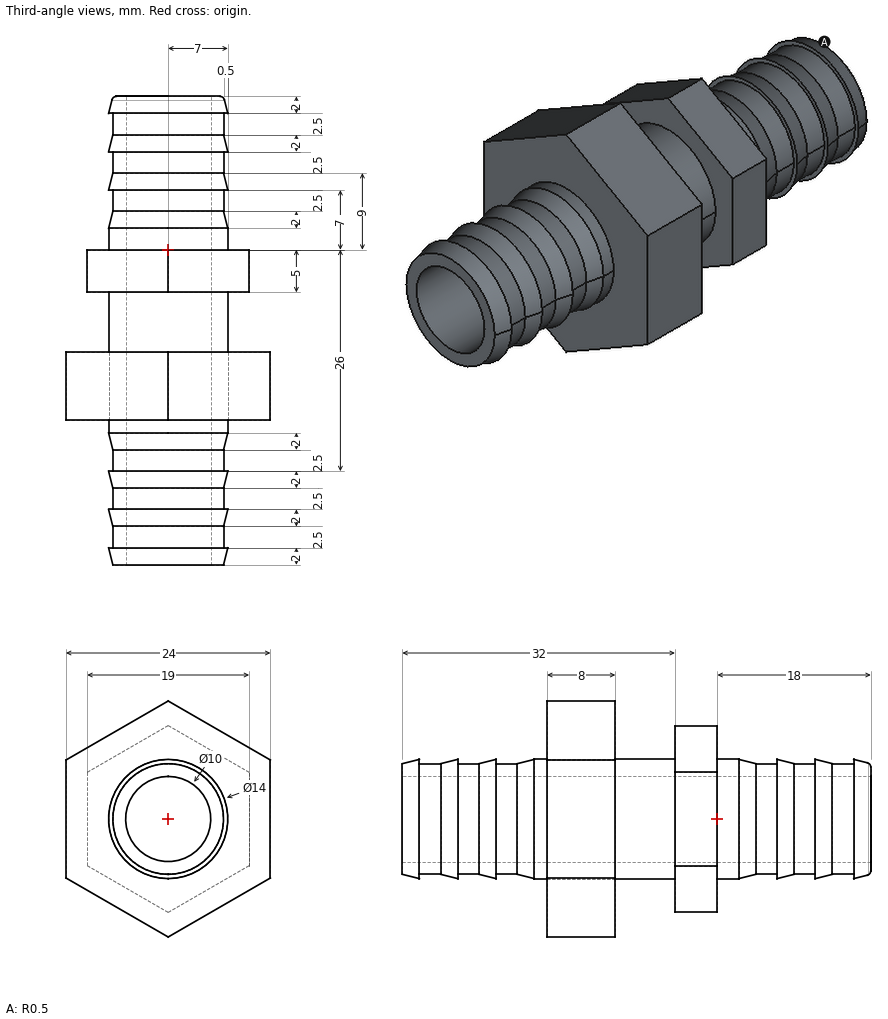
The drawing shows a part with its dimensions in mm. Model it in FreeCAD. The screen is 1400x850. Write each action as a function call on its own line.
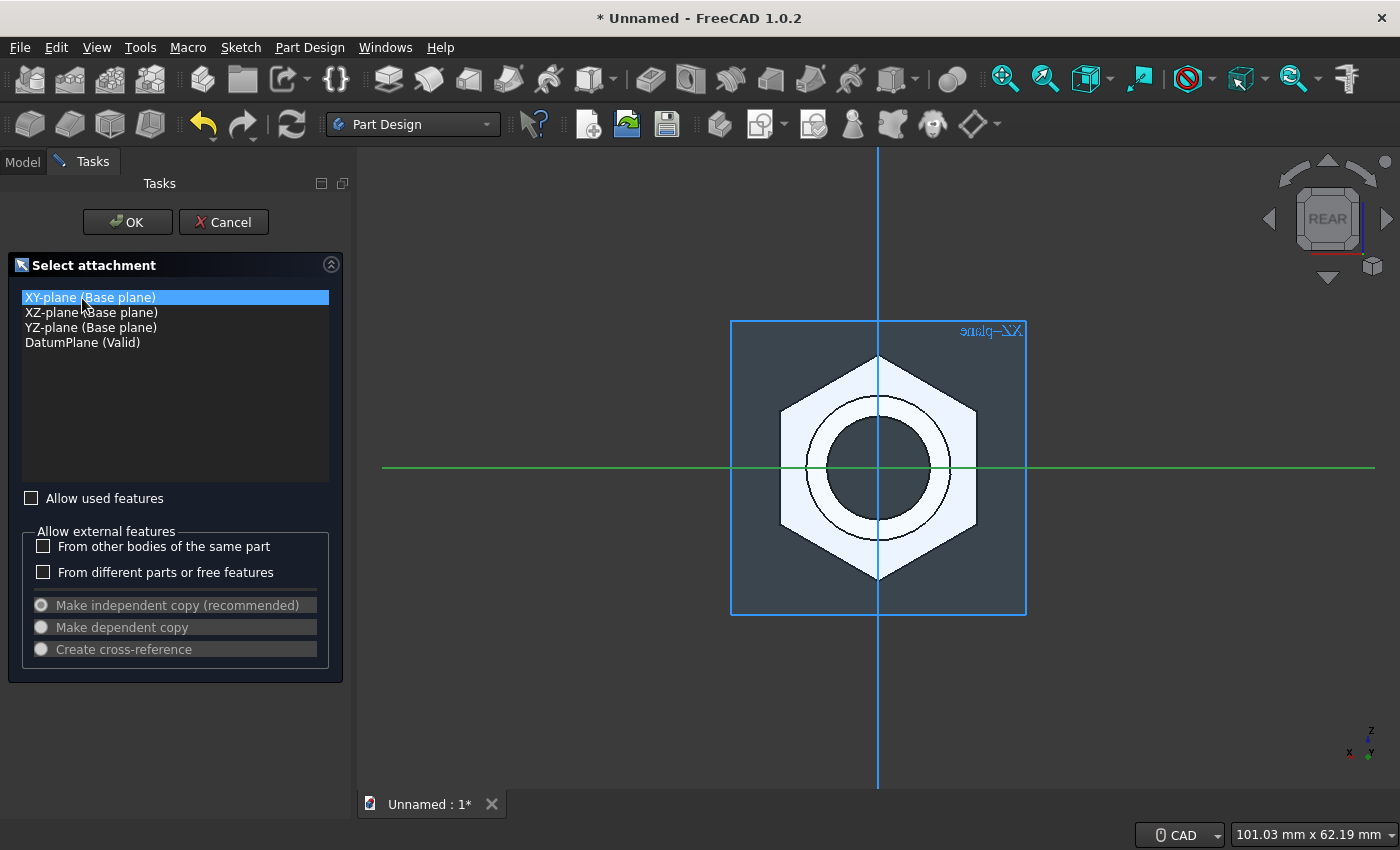
click(128, 222)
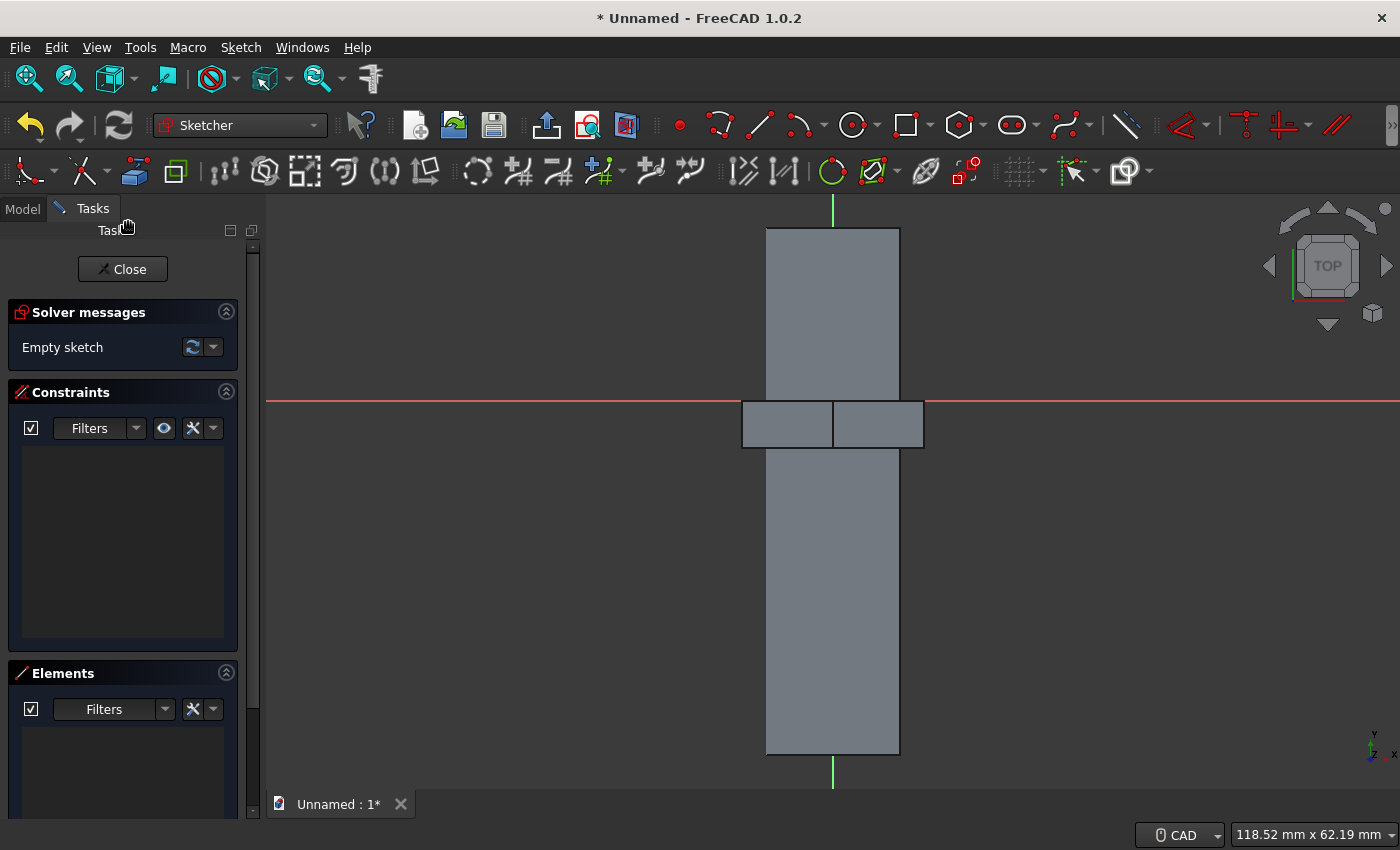
click(628, 126)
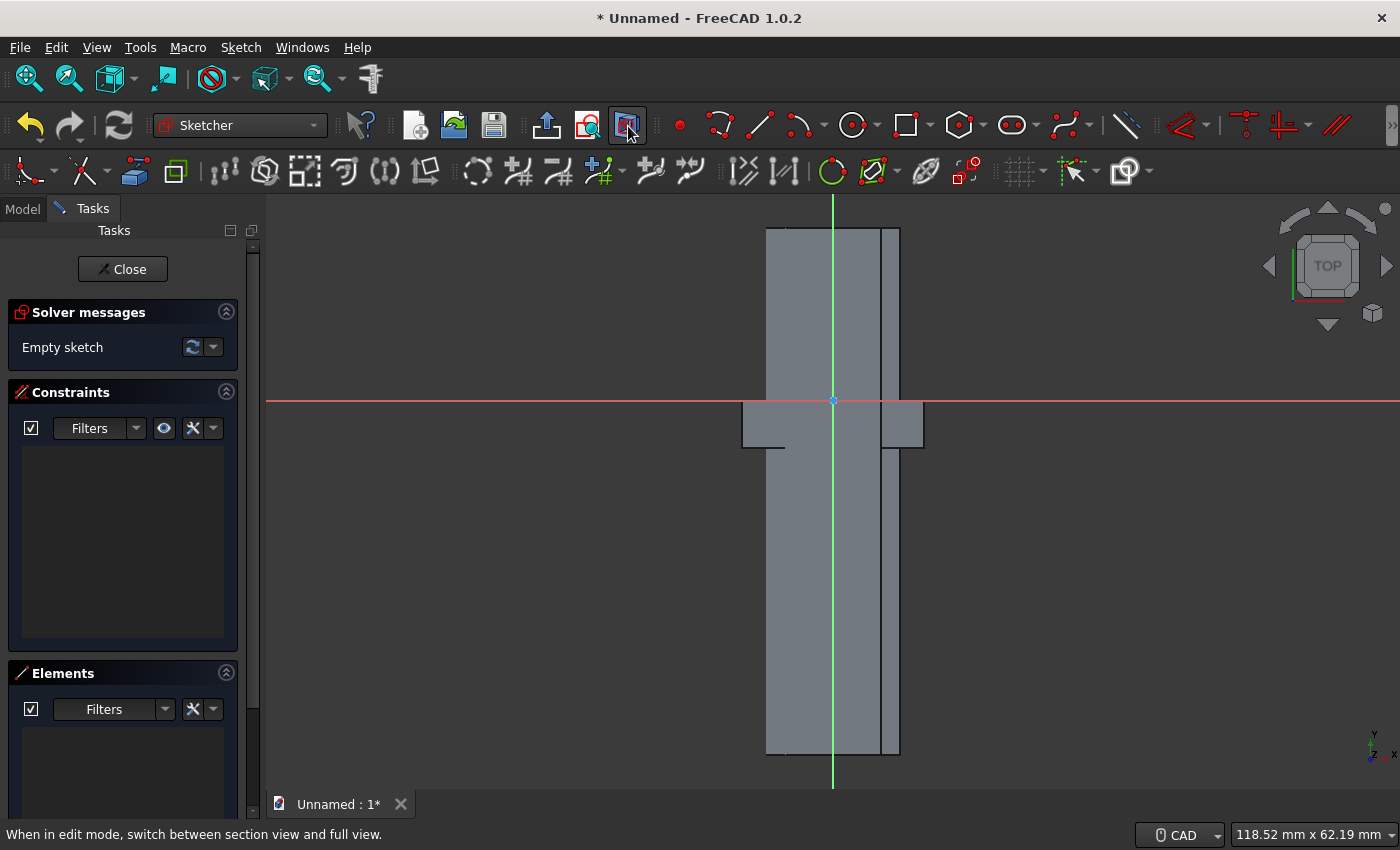
scroll(557, 492, down, 2)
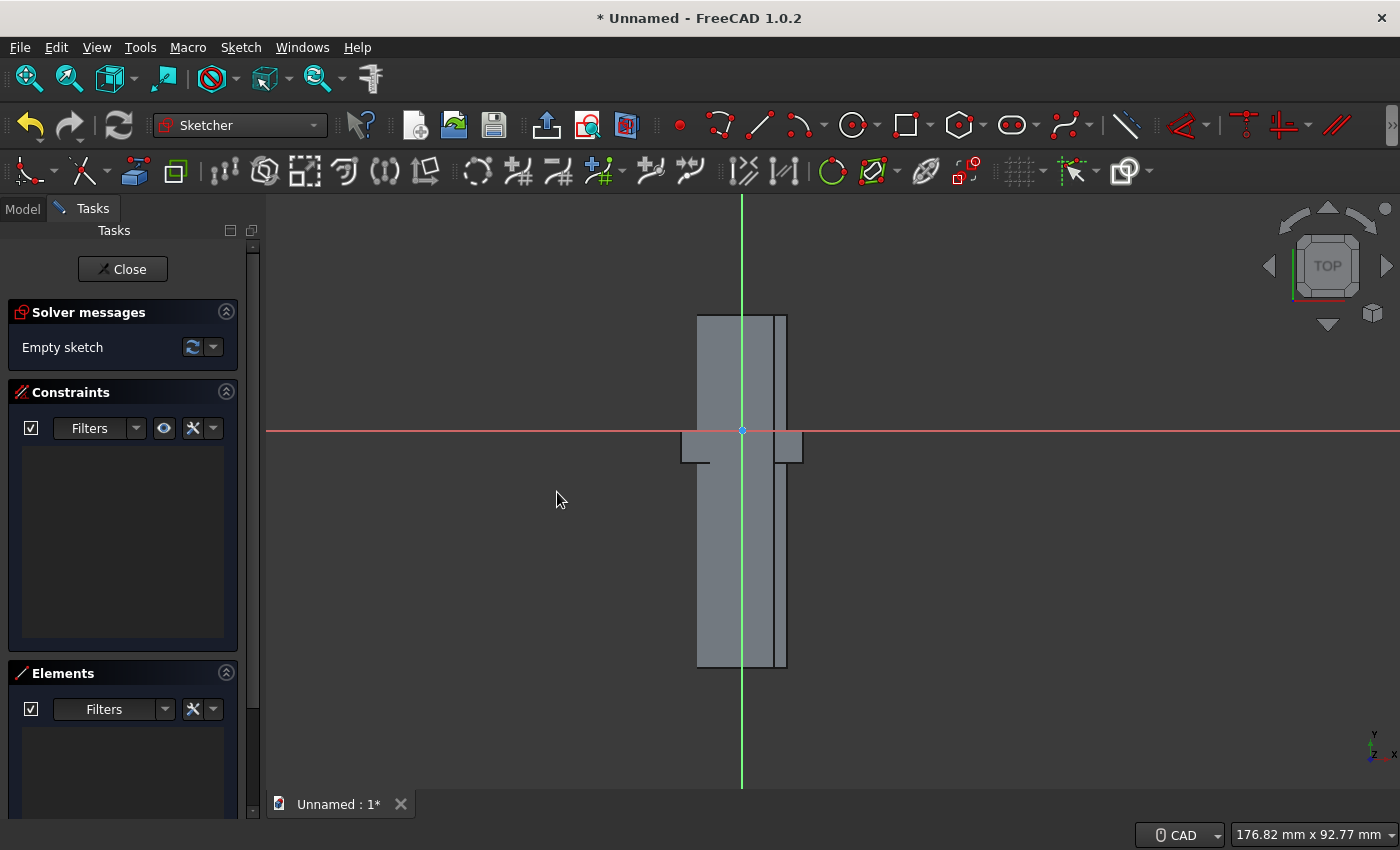
click(720, 126)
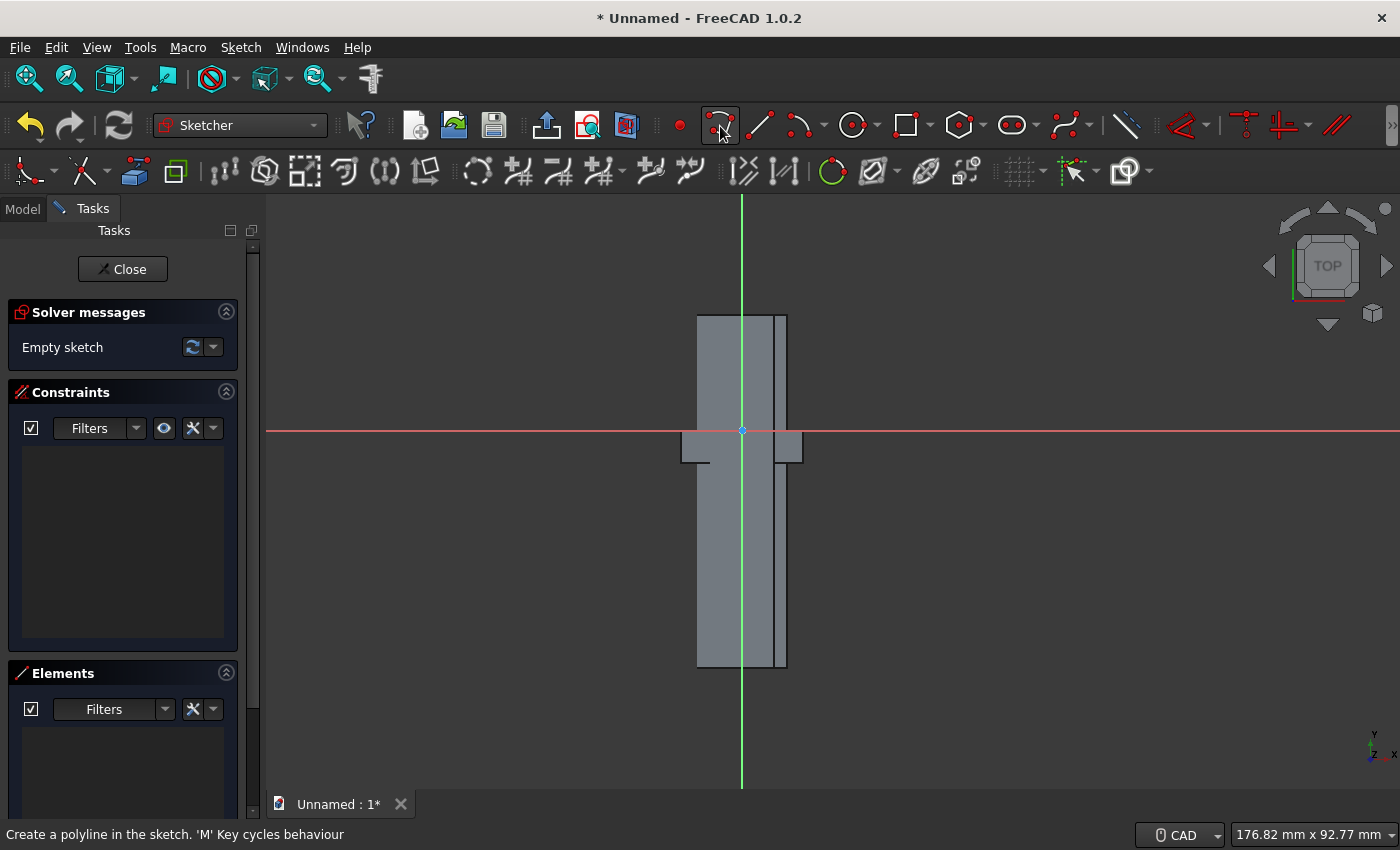
click(787, 415)
click(787, 315)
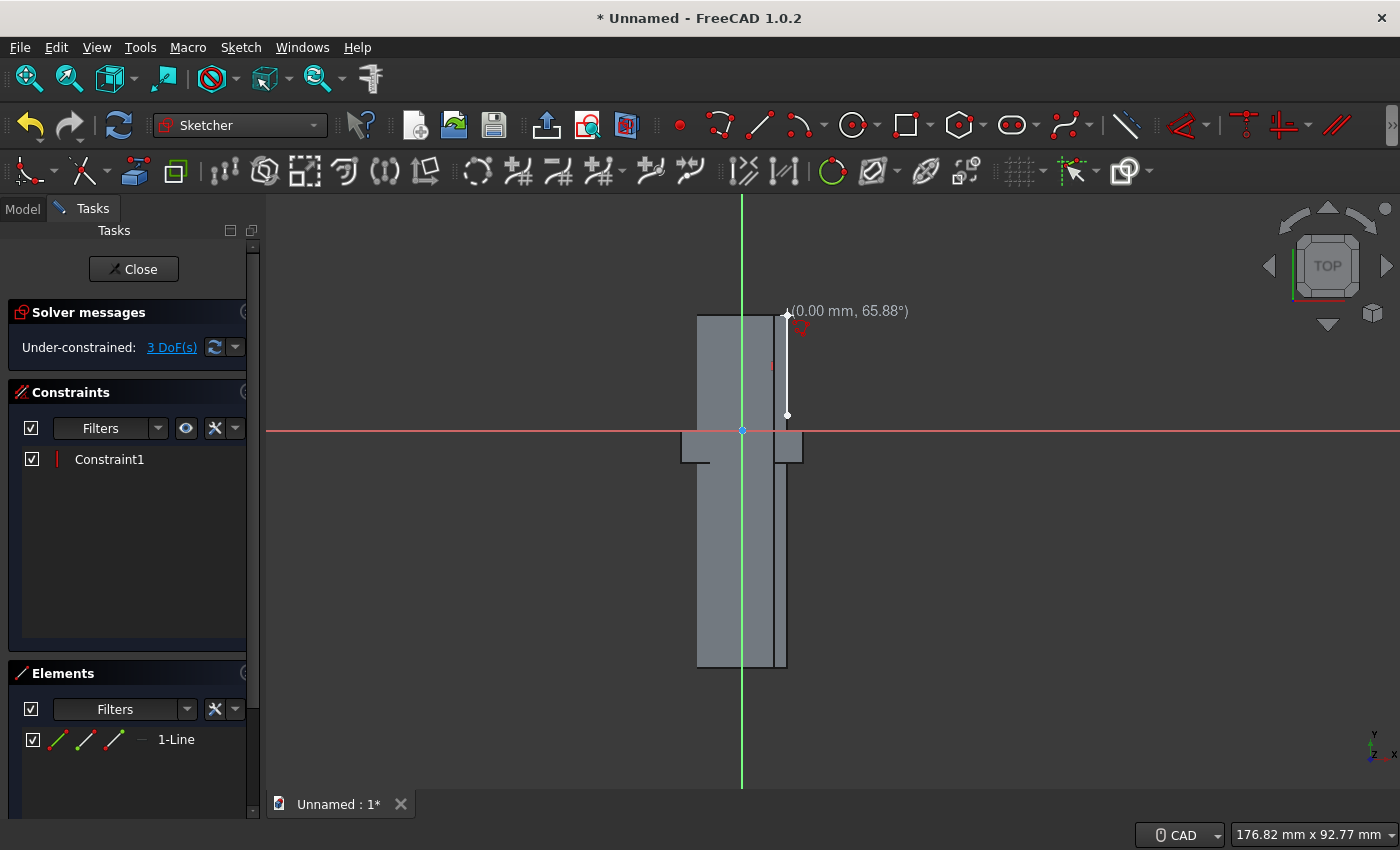
scroll(784, 315, up, 8)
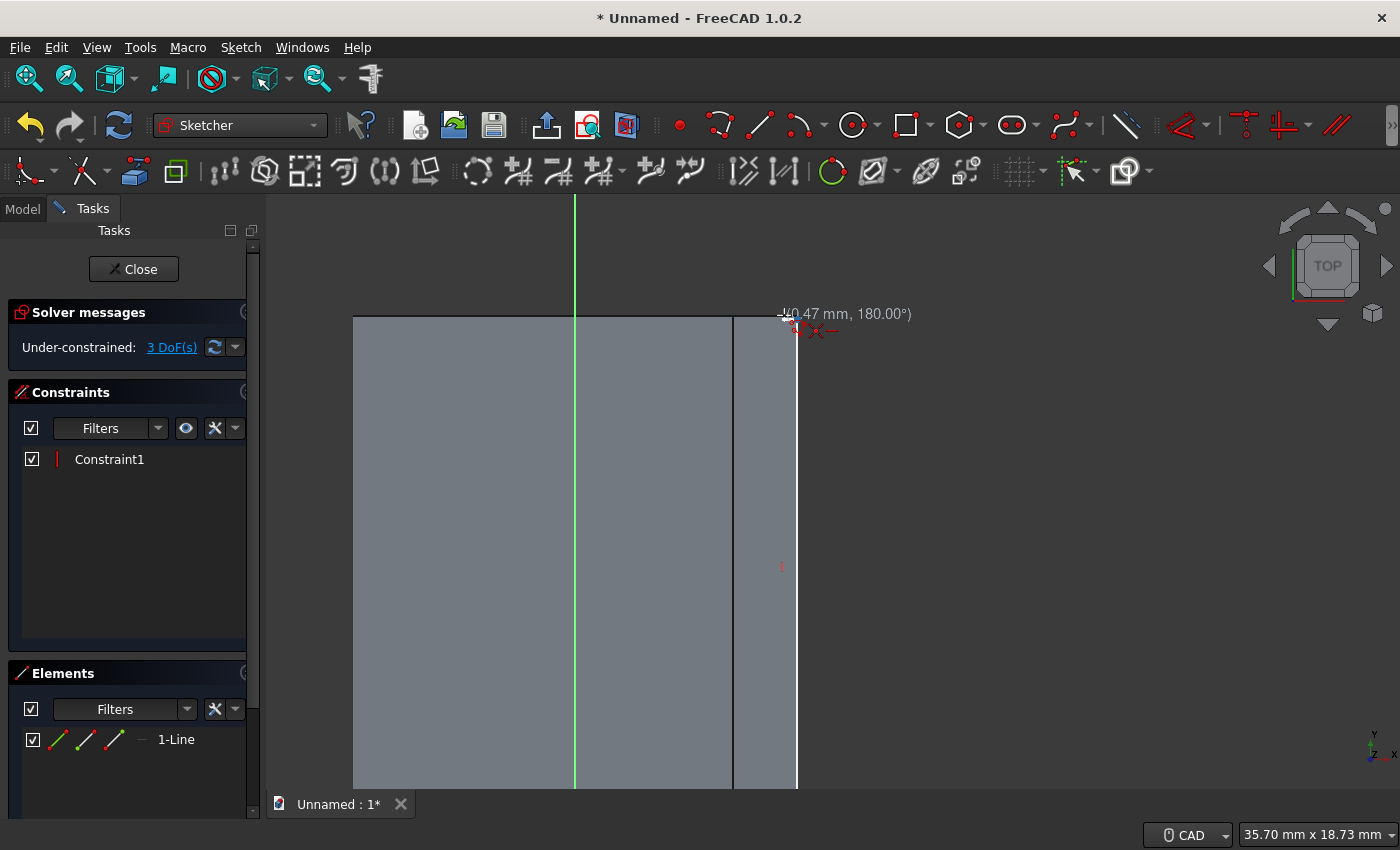
click(781, 314)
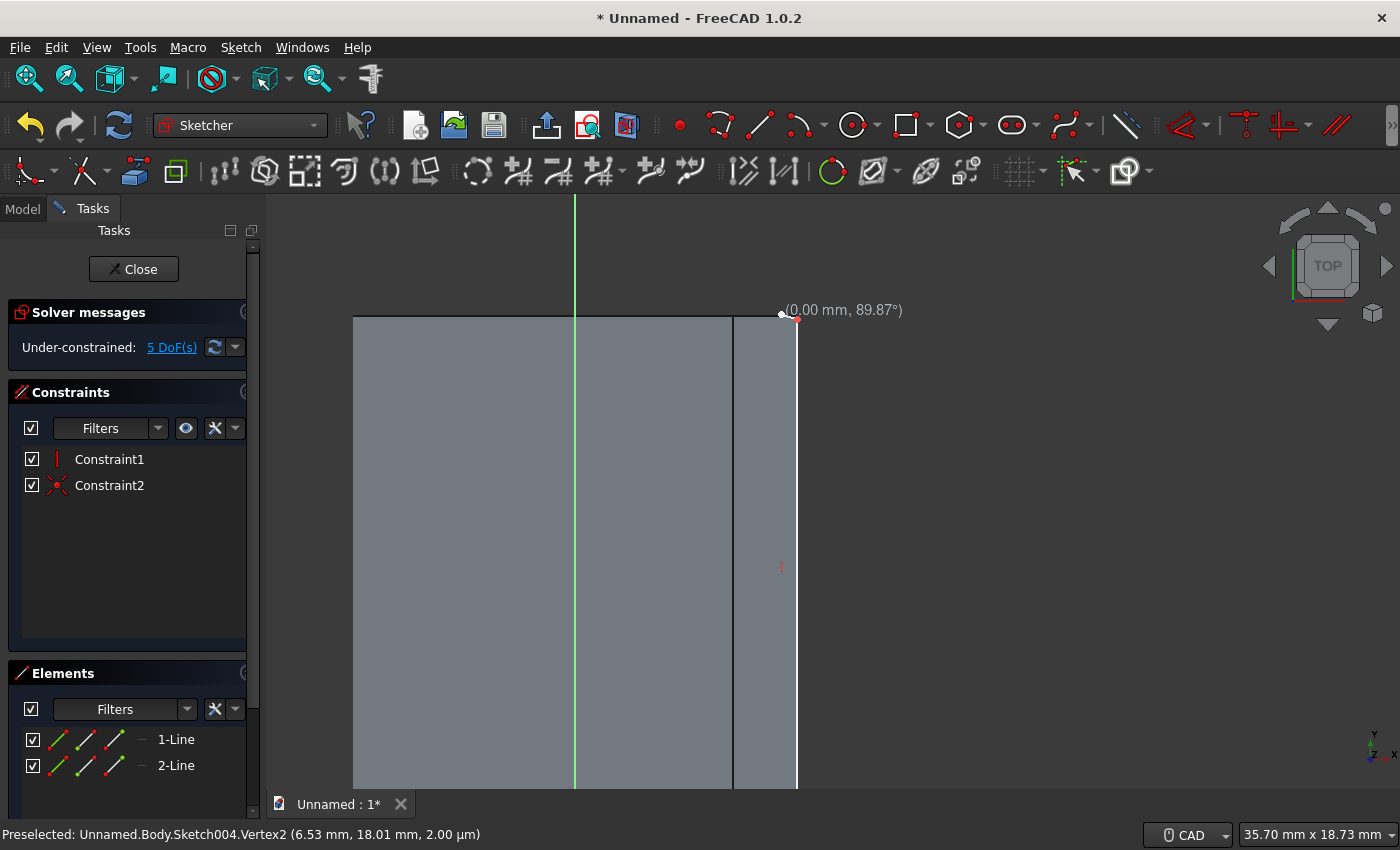
scroll(784, 315, down, 8)